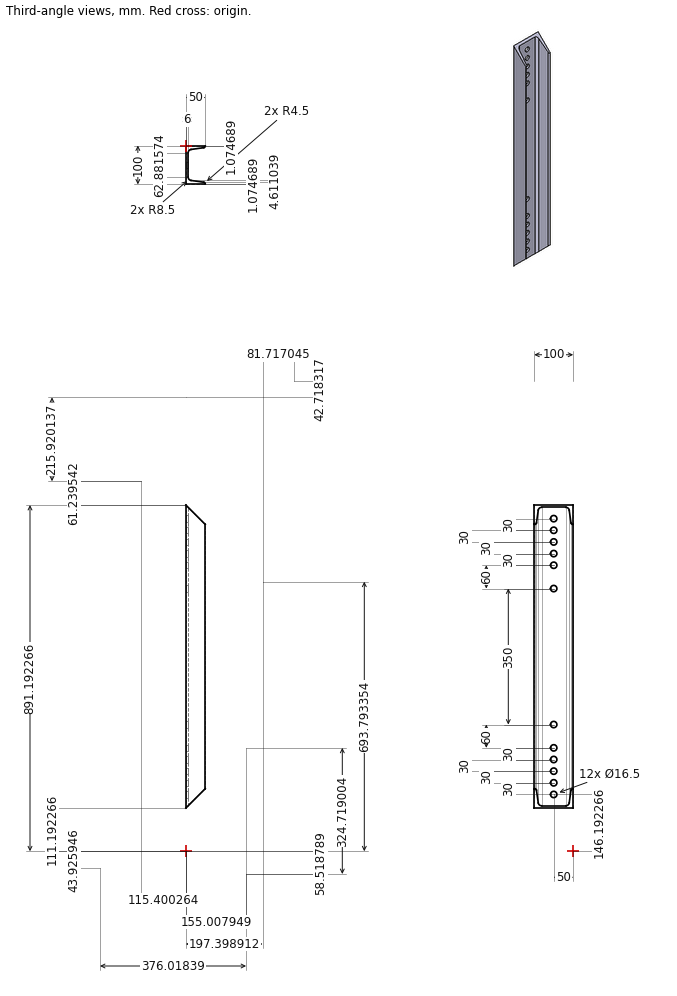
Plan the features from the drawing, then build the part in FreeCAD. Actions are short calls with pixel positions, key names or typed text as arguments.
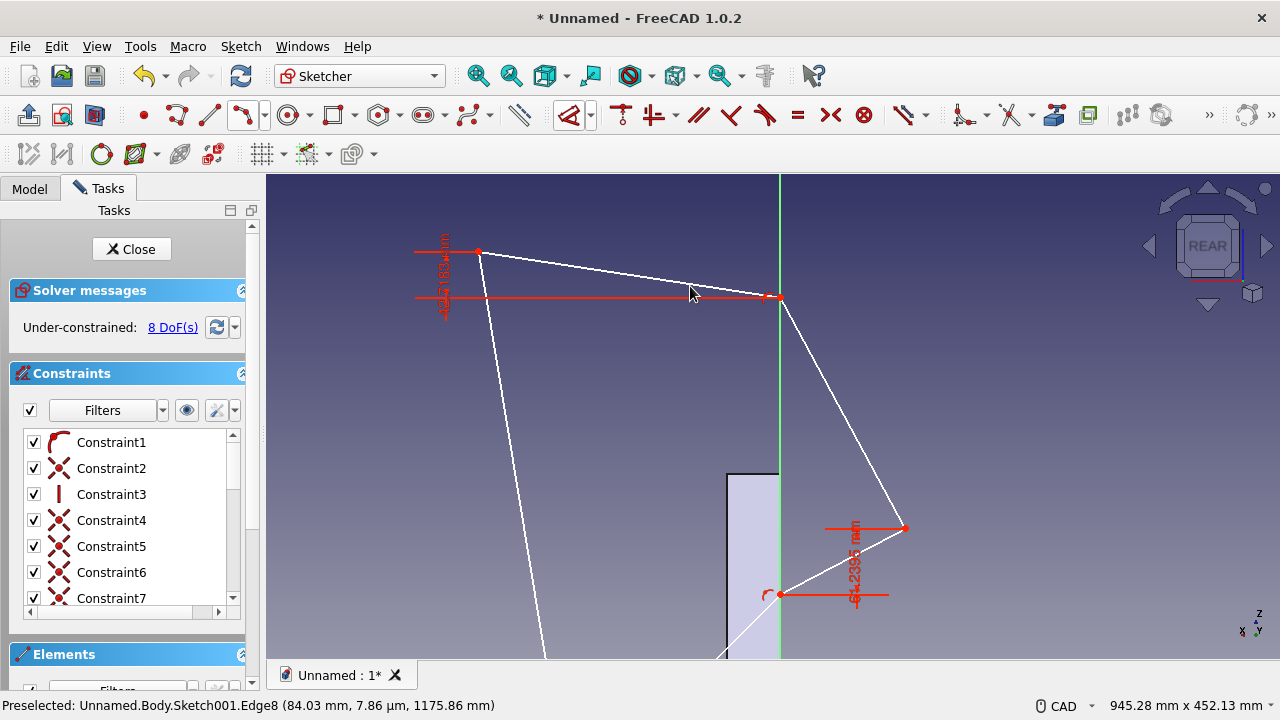
click(506, 419)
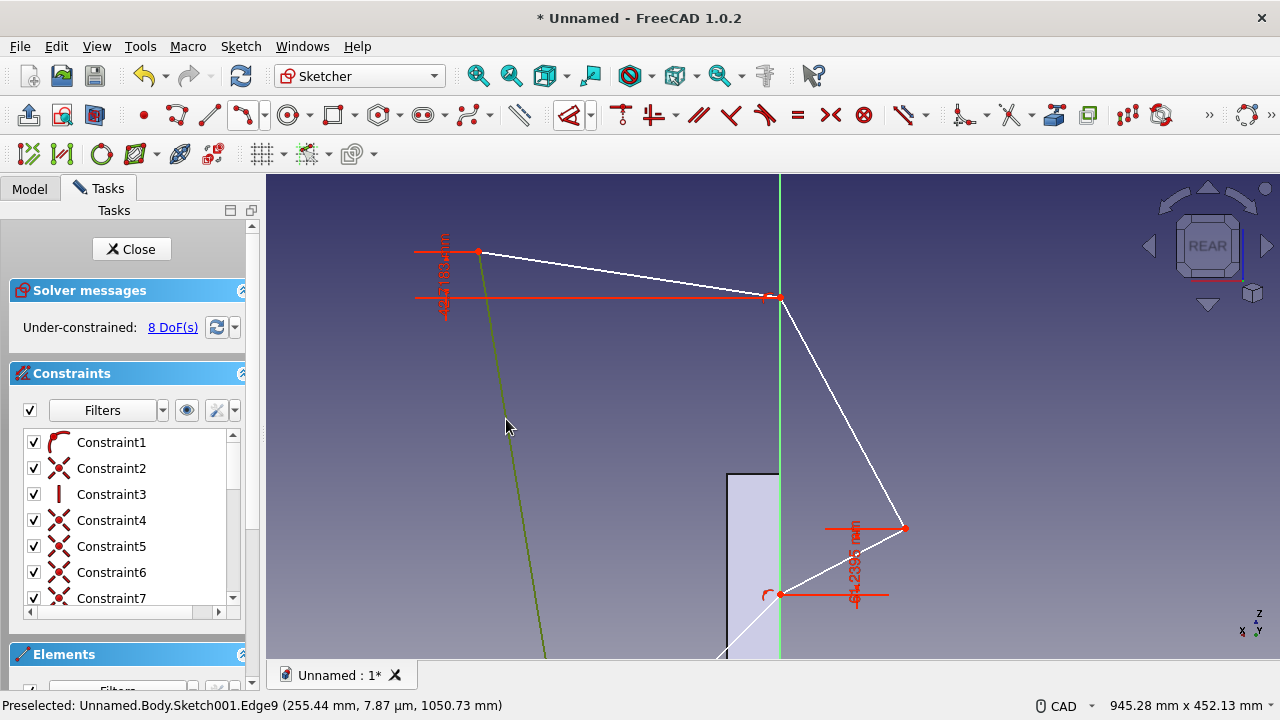
click(590, 116)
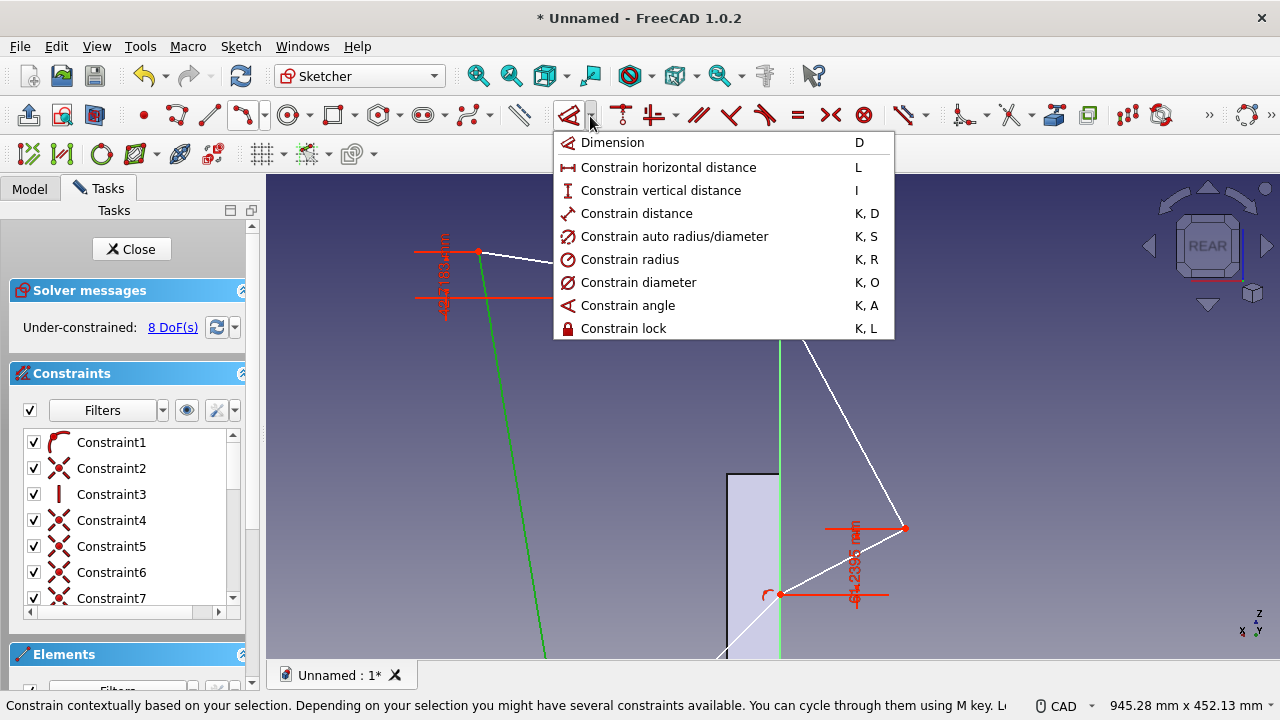
click(724, 168)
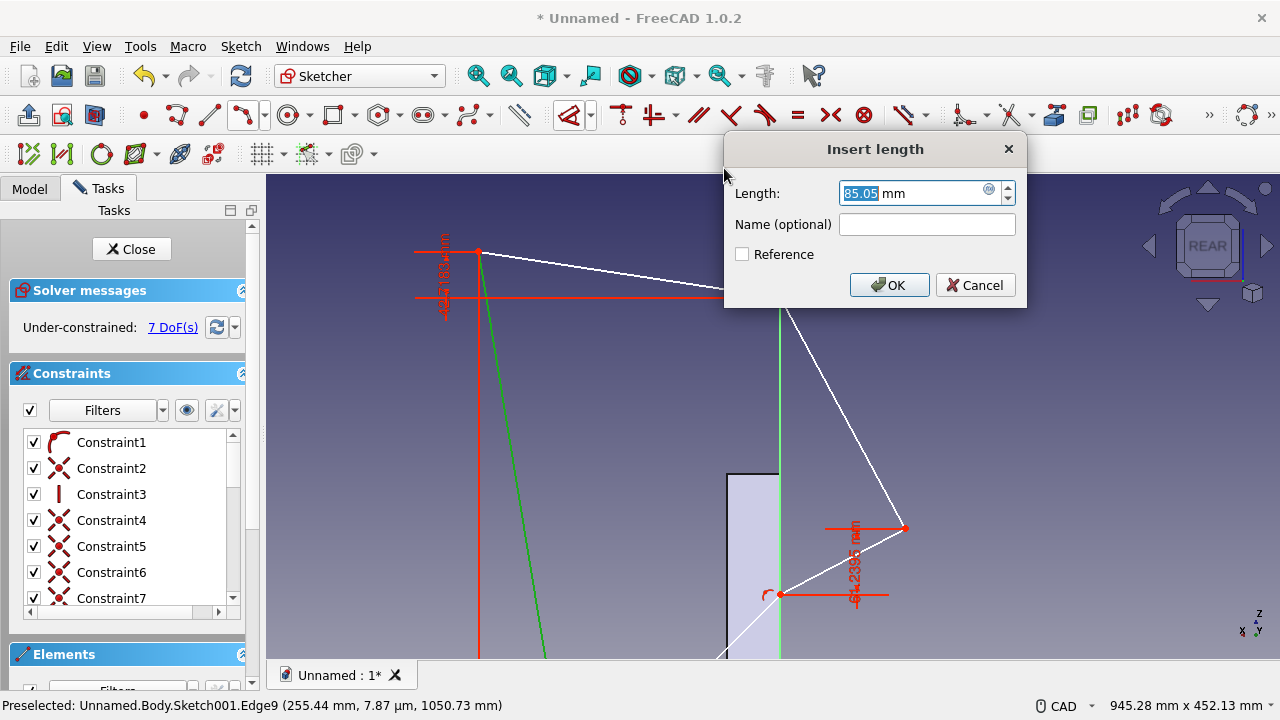
text(81.717045)
key(Return)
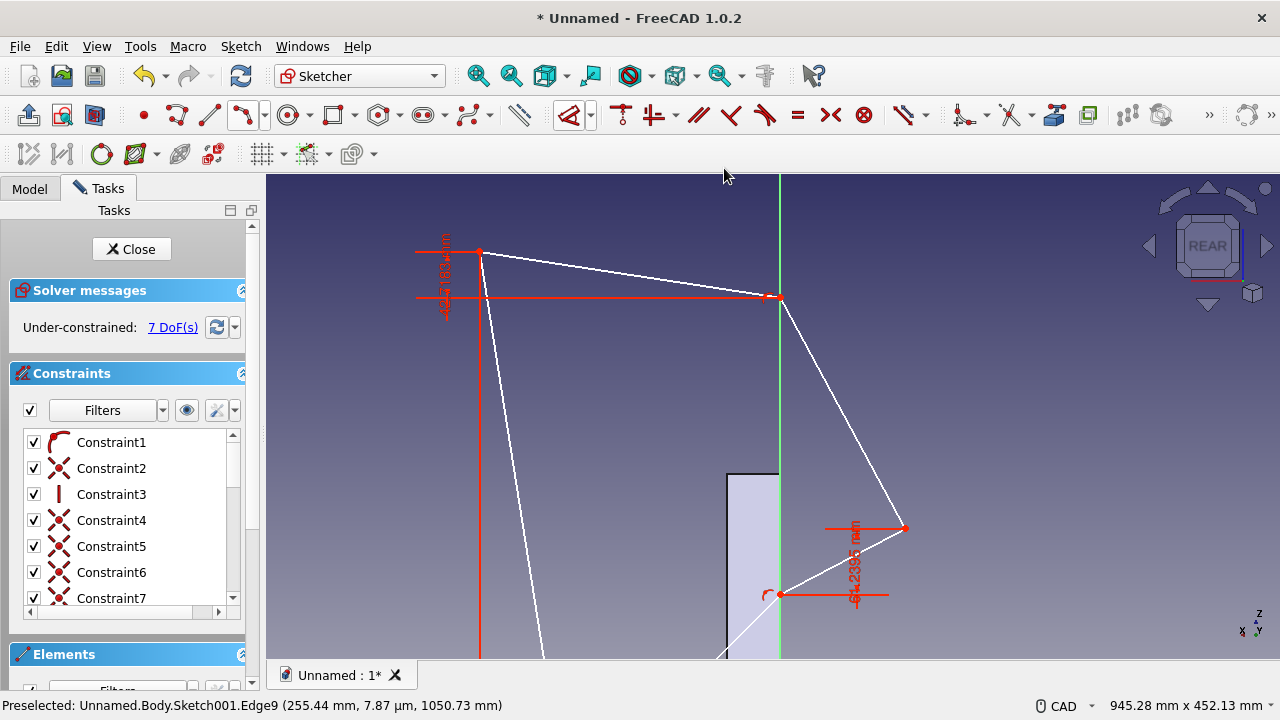
scroll(693, 287, down, 8)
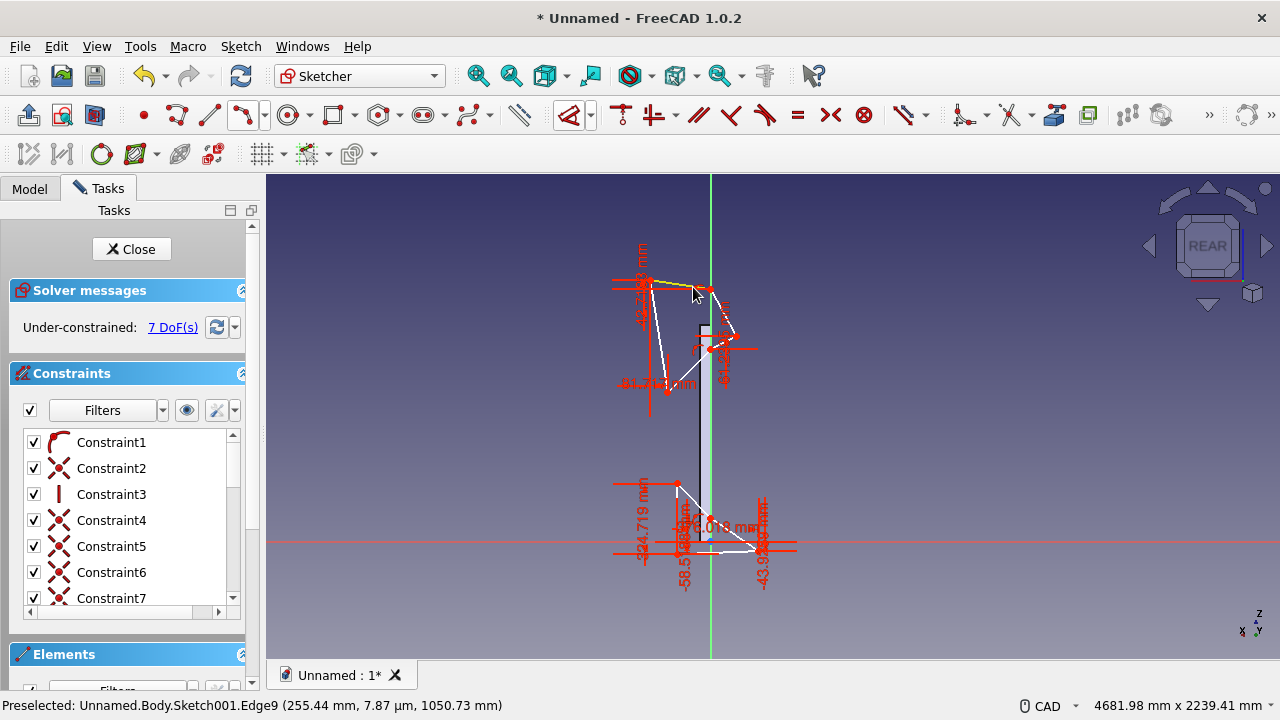
scroll(711, 518, up, 3)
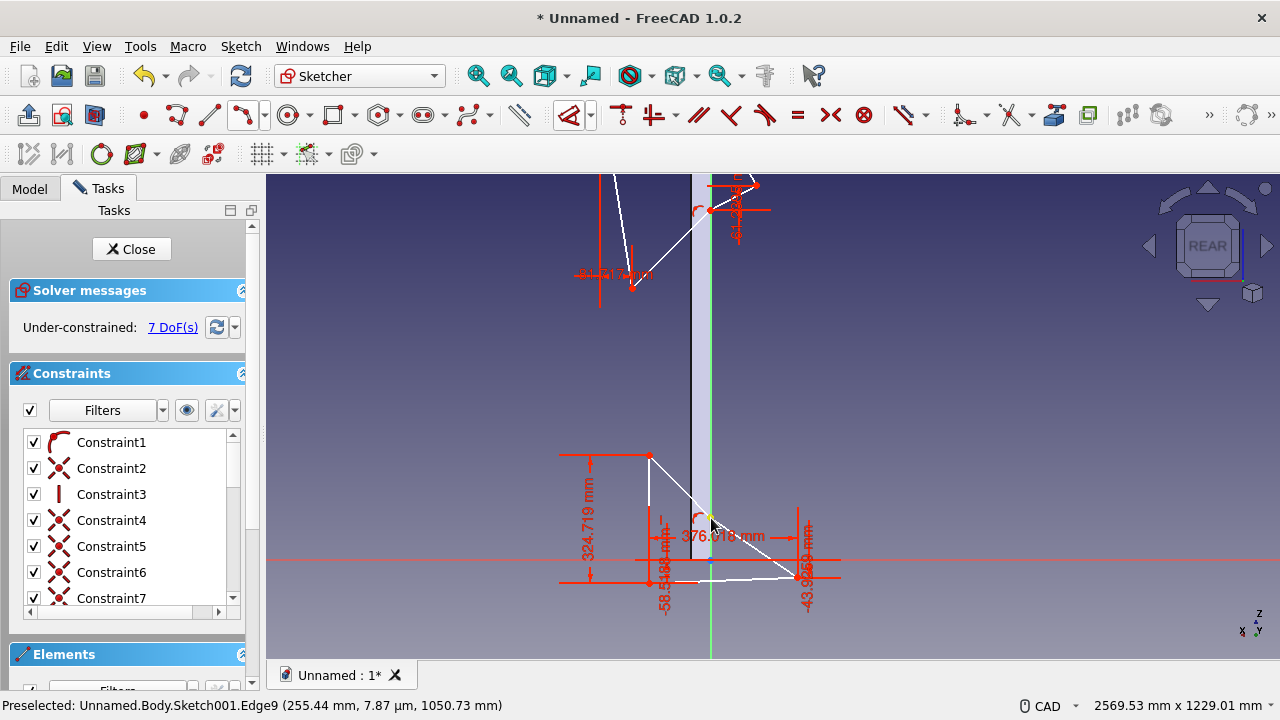
click(711, 518)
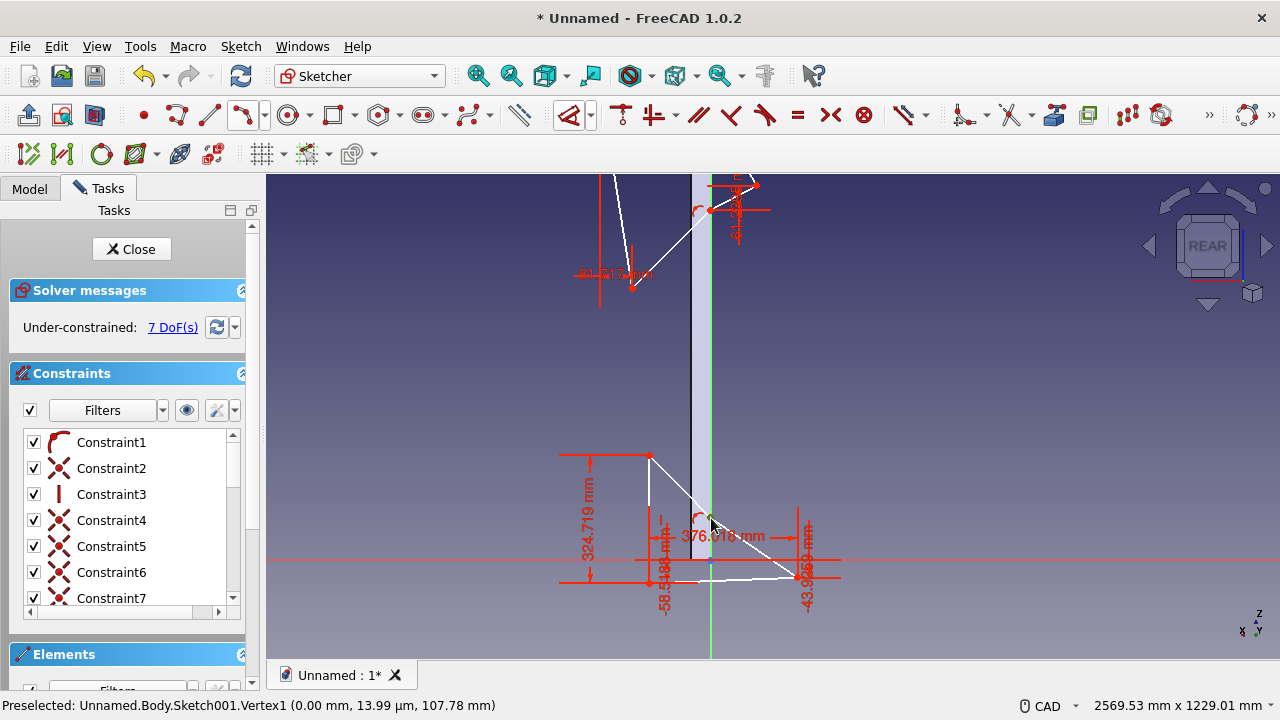
key(i)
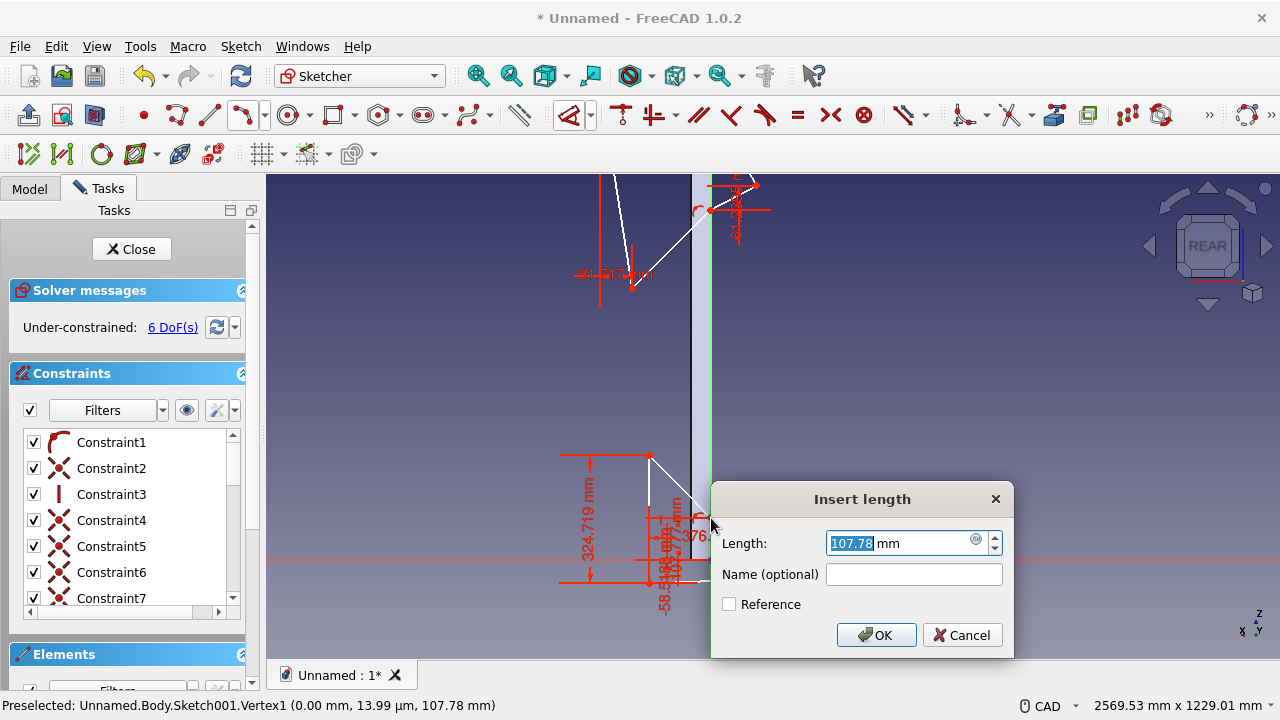
text(111.192266)
key(Return)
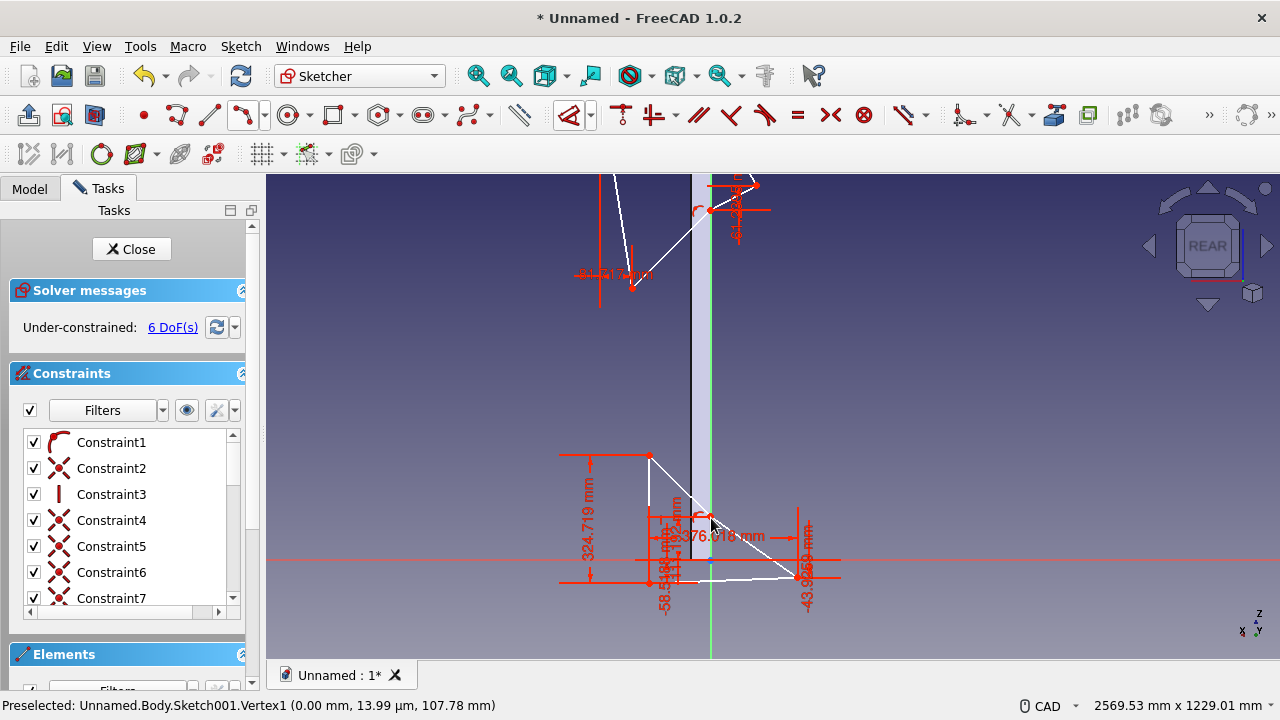
click(649, 455)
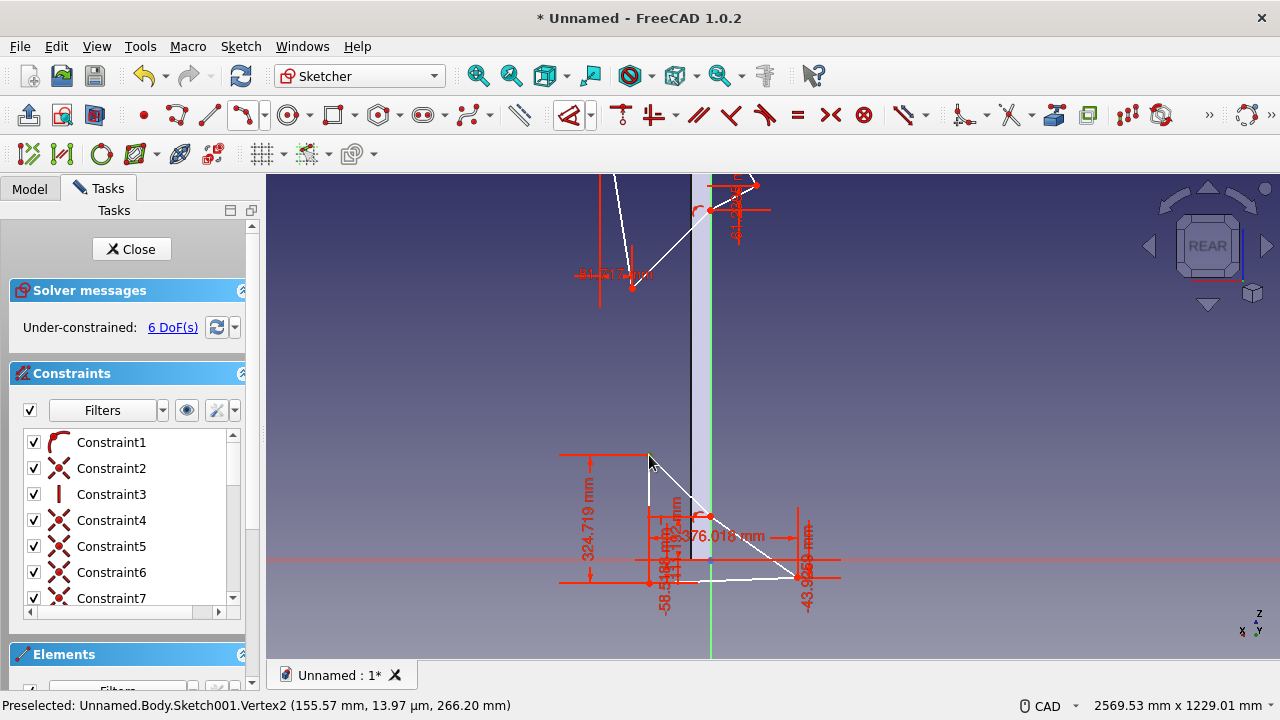
click(590, 116)